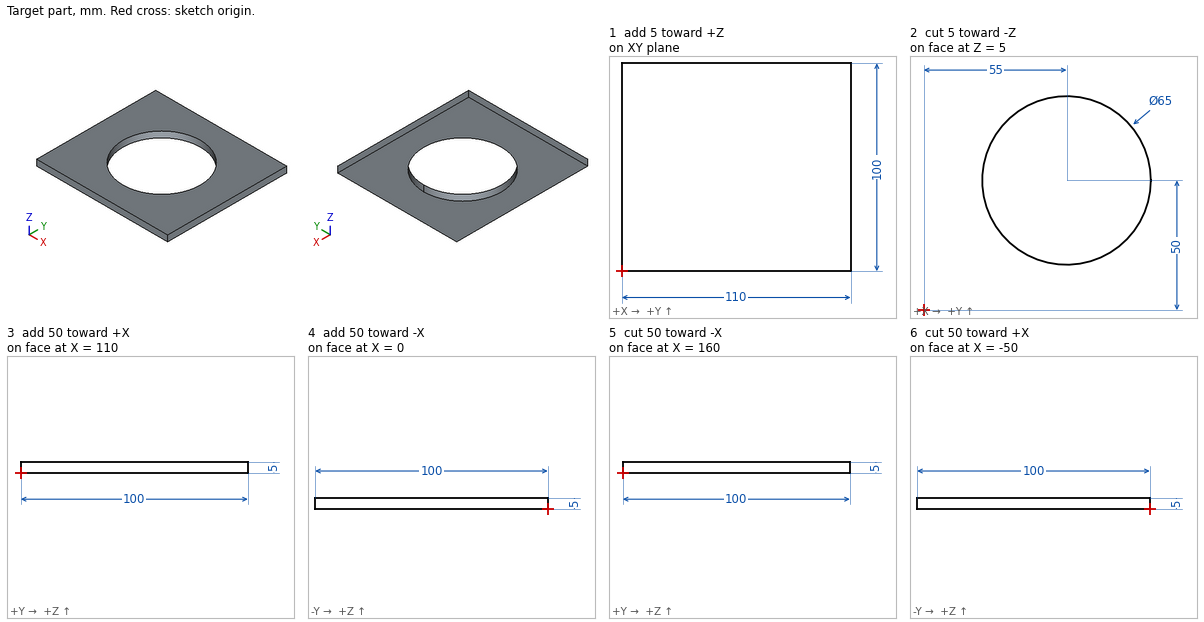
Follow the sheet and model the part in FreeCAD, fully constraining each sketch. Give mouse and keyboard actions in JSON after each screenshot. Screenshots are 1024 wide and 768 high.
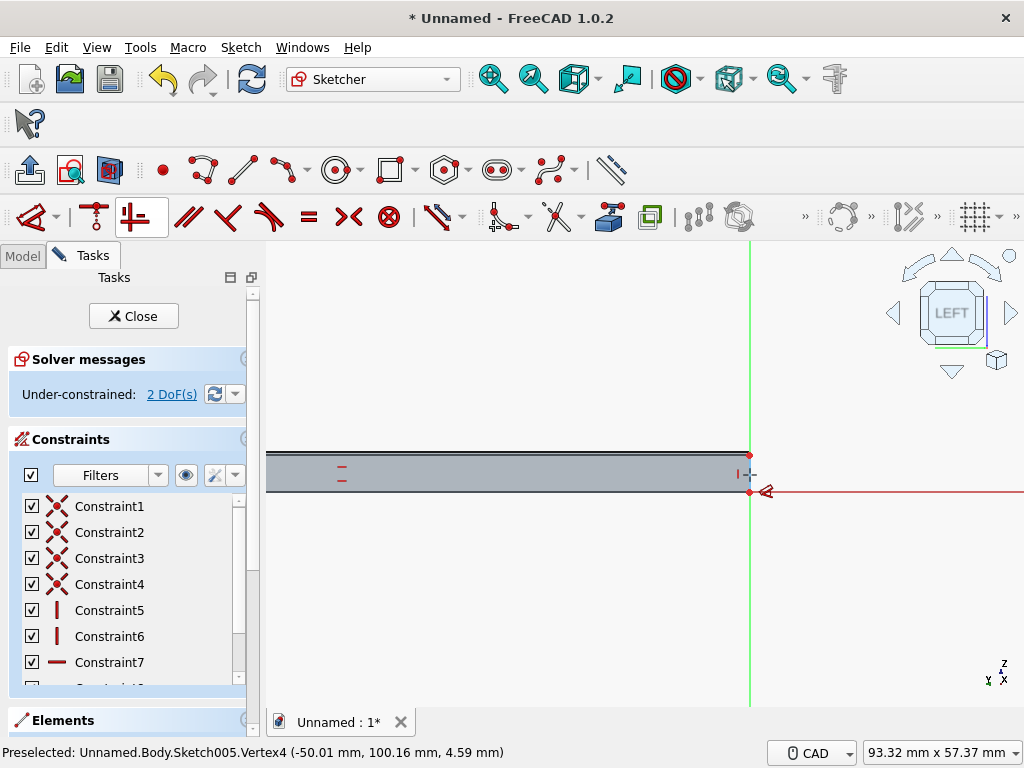
{"action": "left_click", "coordinate": [750, 474]}
{"action": "left_click", "coordinate": [784, 474]}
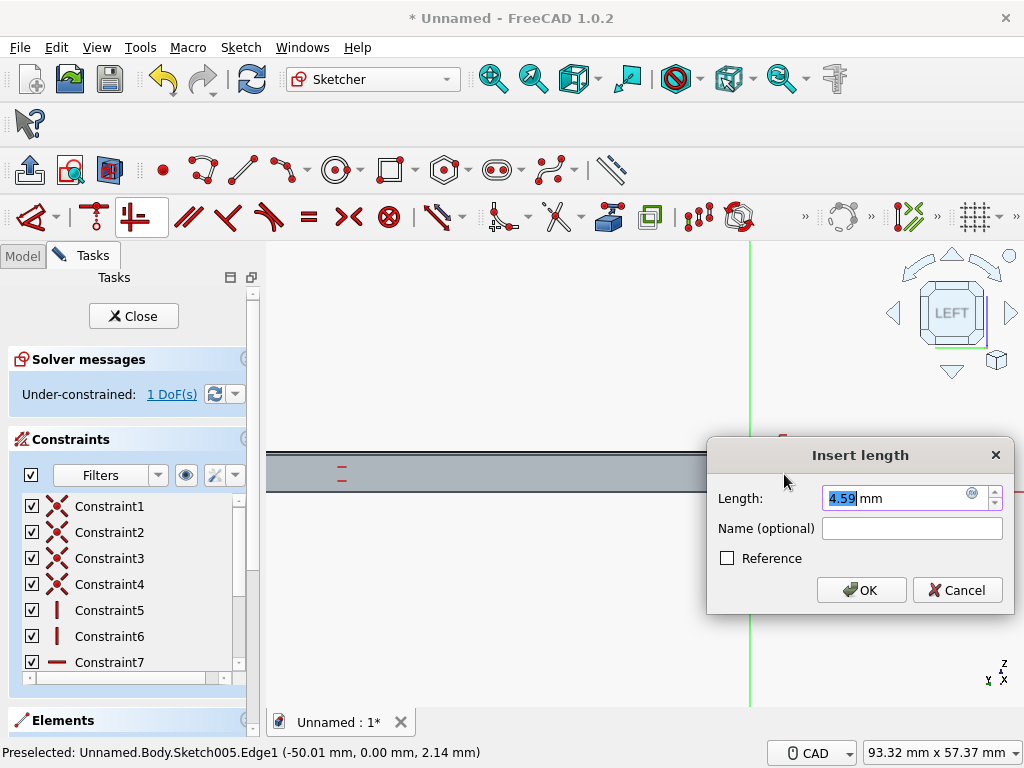
{"action": "type", "text": "5"}
{"action": "key", "text": "Return"}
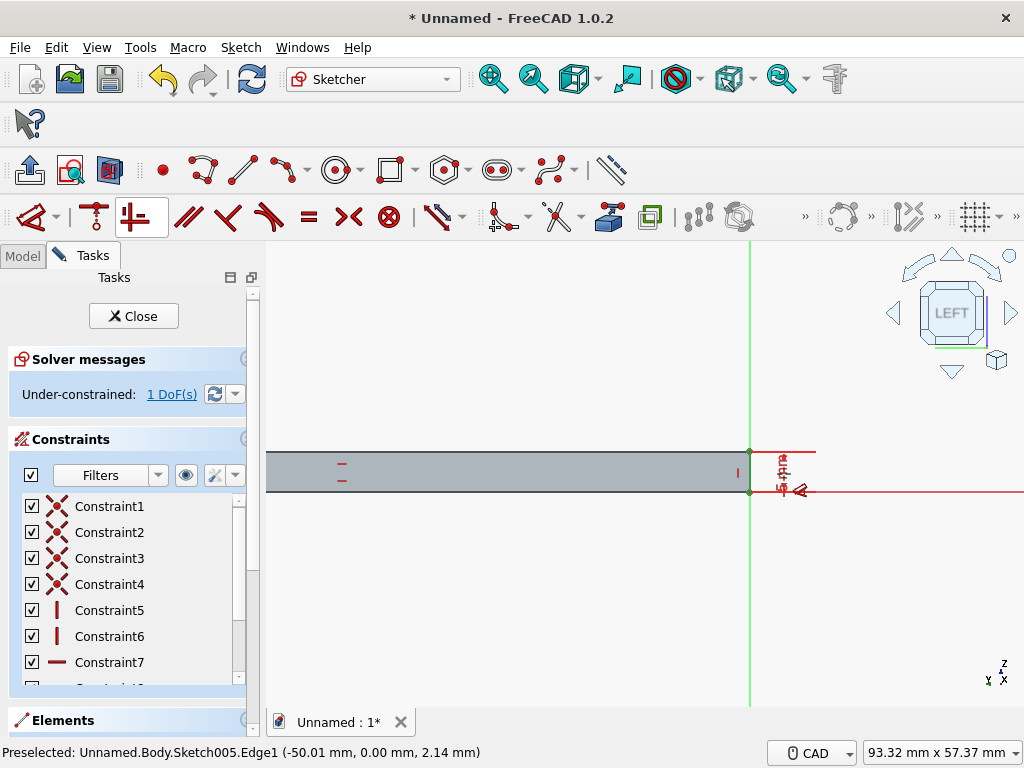
{"action": "left_click", "coordinate": [506, 452]}
{"action": "left_click", "coordinate": [522, 418]}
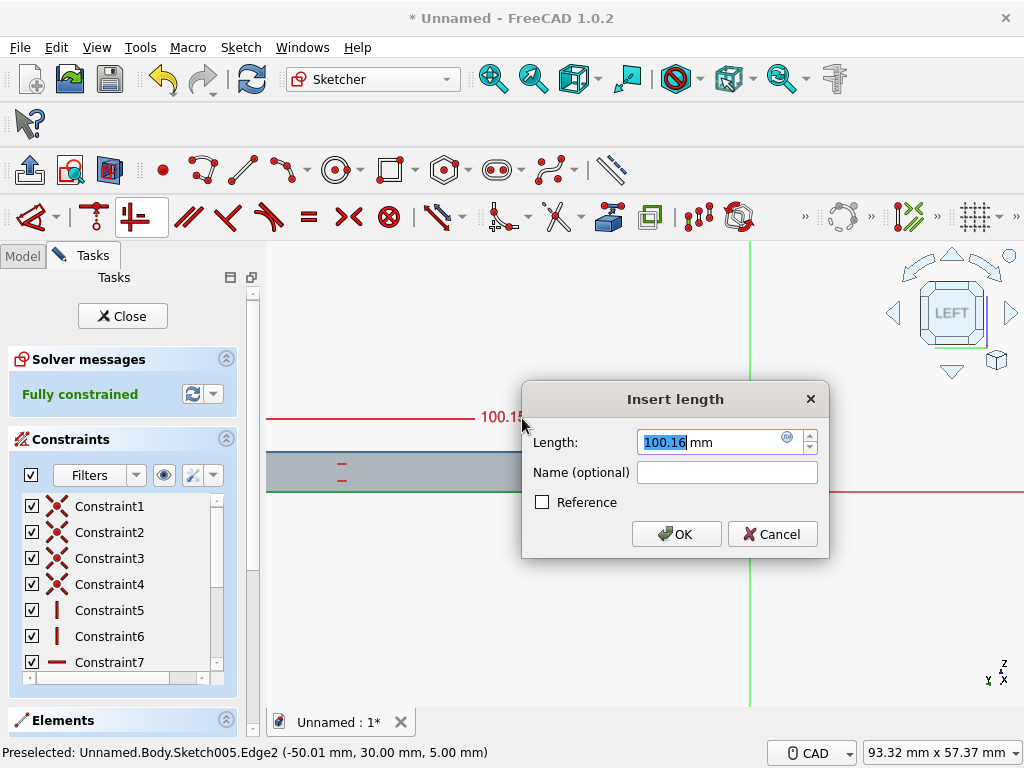
{"action": "type", "text": "100"}
{"action": "key", "text": "Return"}
{"action": "key", "text": "Escape"}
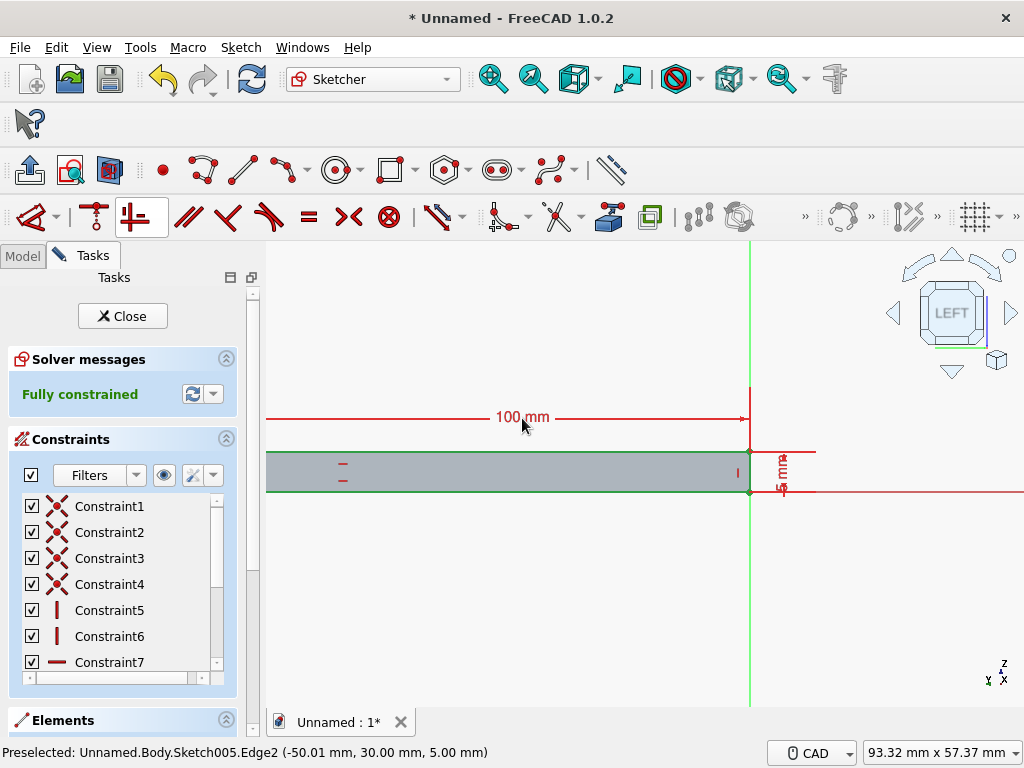
{"action": "left_click", "coordinate": [123, 316]}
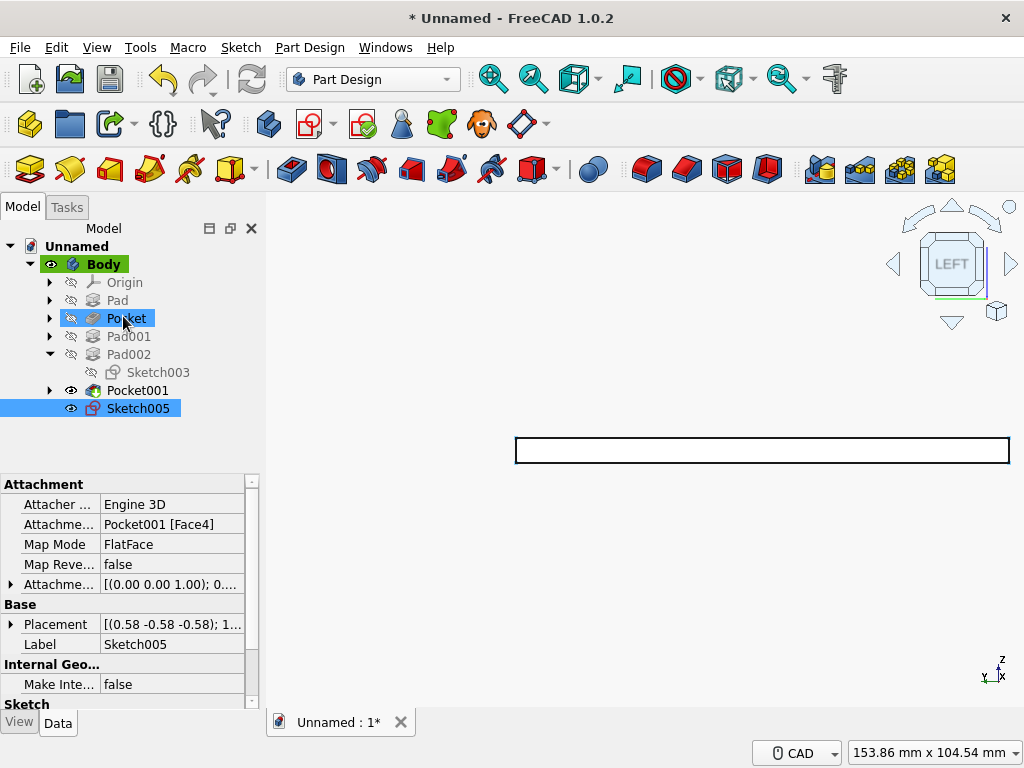
{"action": "left_click", "coordinate": [292, 170]}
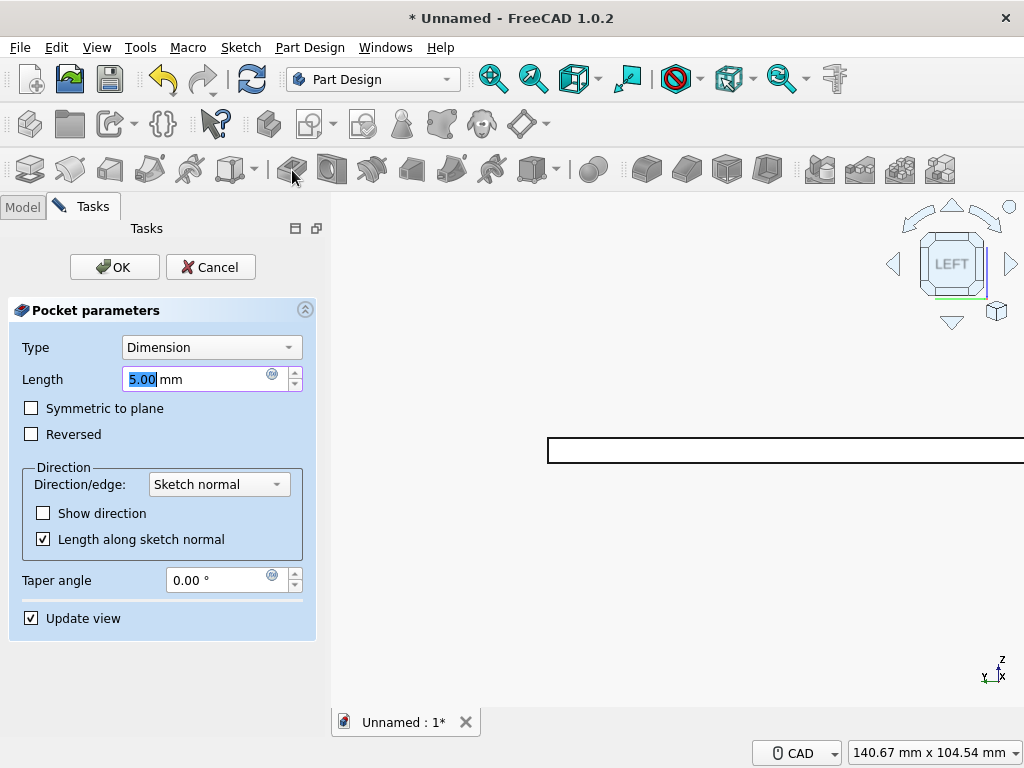
{"action": "type", "text": "50"}
{"action": "key", "text": "Tab"}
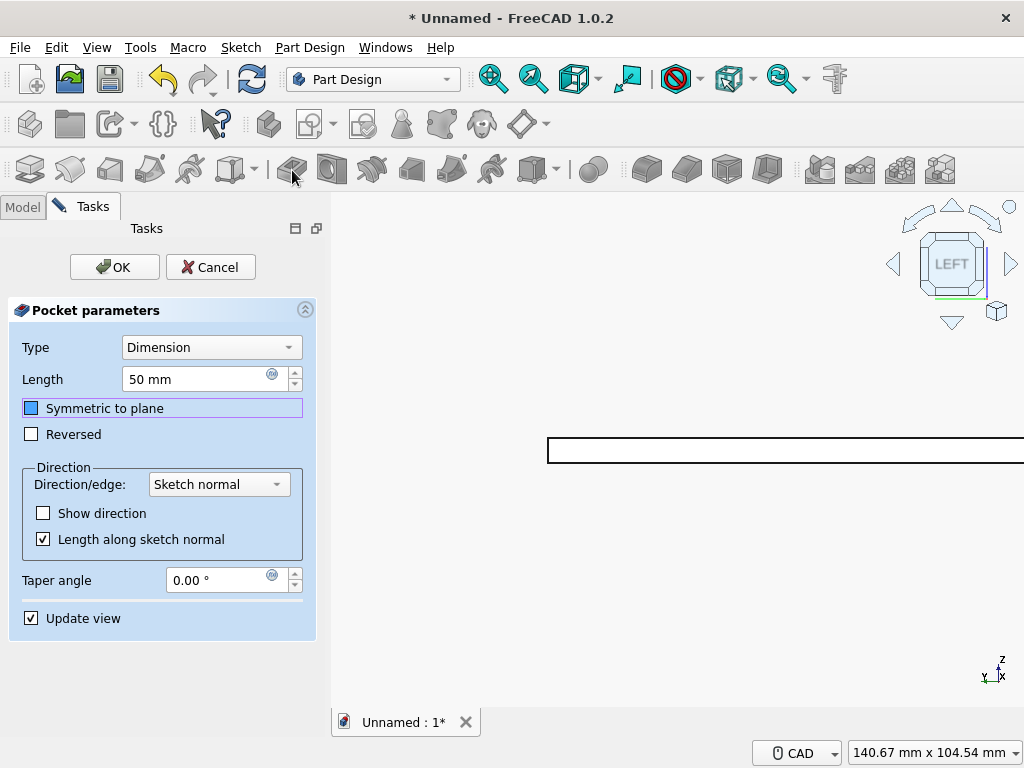
{"action": "left_click", "coordinate": [115, 267]}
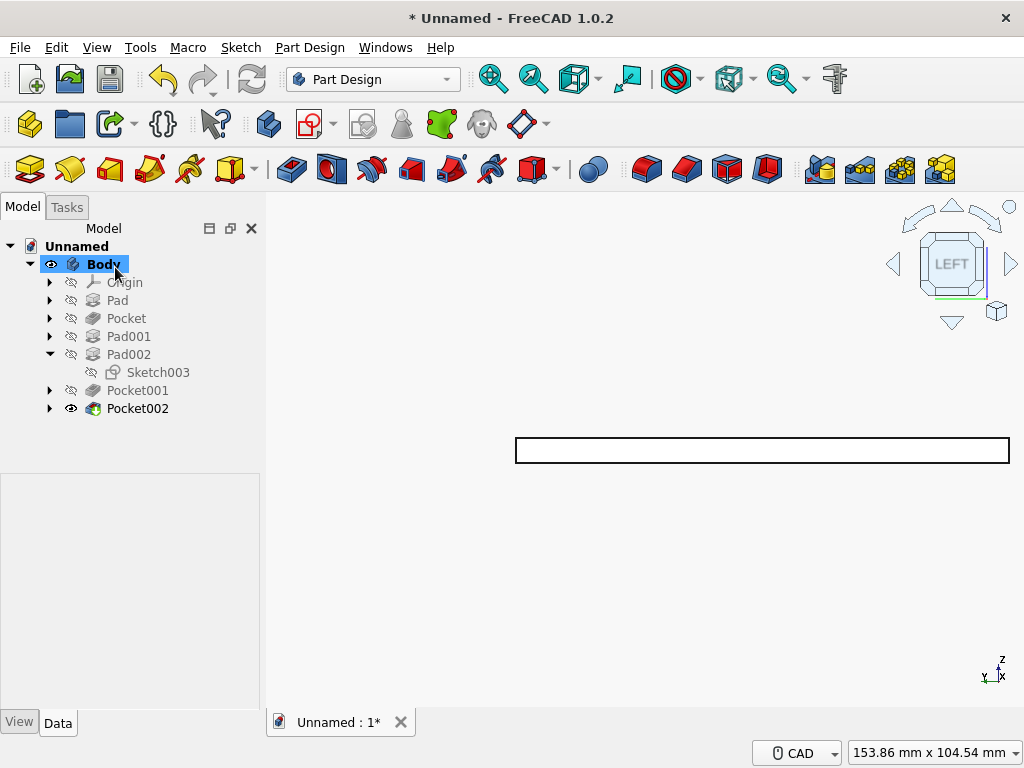
{"action": "key", "text": "0"}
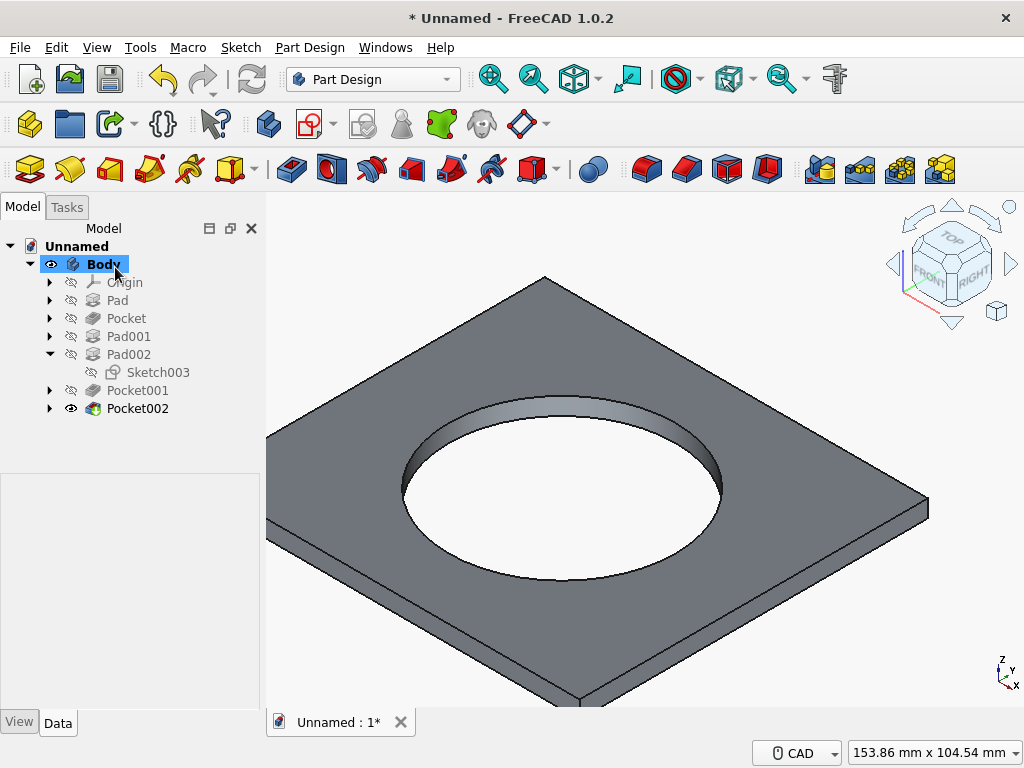
{"action": "left_click", "coordinate": [494, 80]}